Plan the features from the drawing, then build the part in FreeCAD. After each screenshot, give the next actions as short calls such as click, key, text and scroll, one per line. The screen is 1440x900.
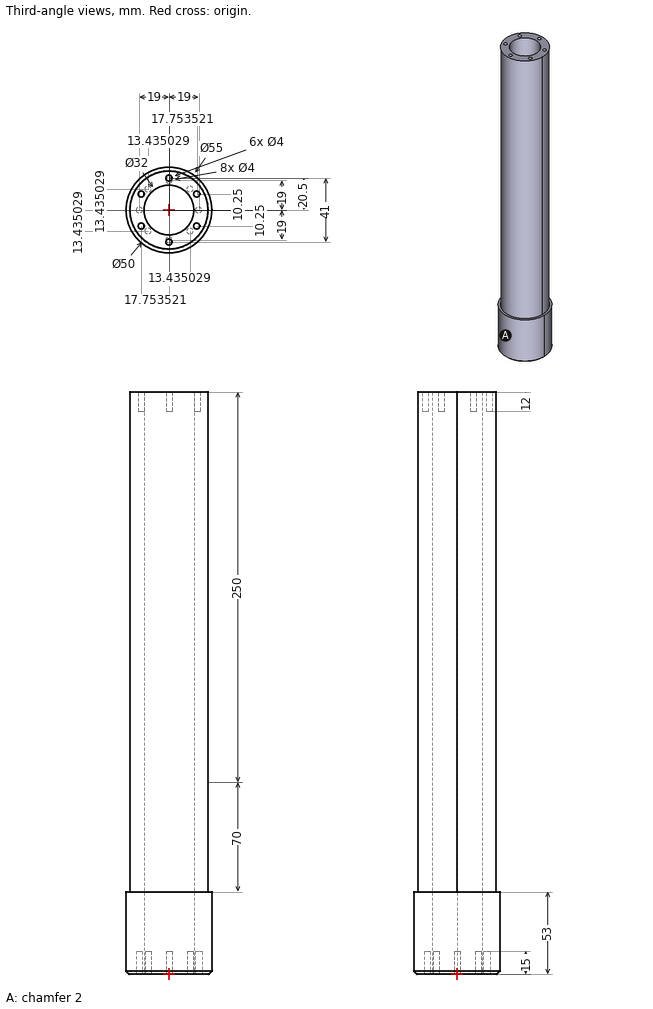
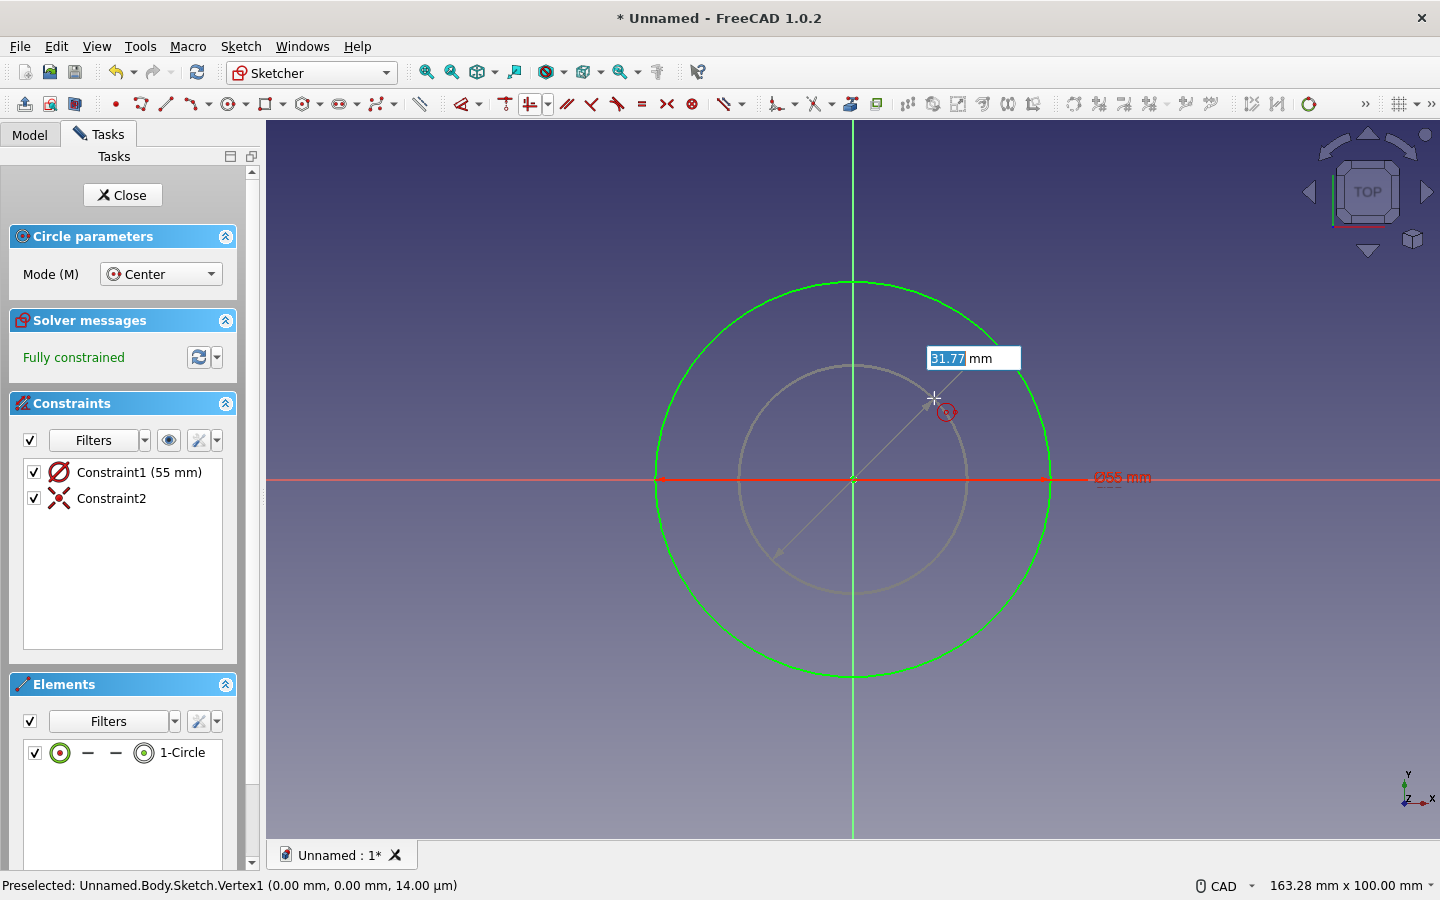
text(32)
key(Return)
key(Escape)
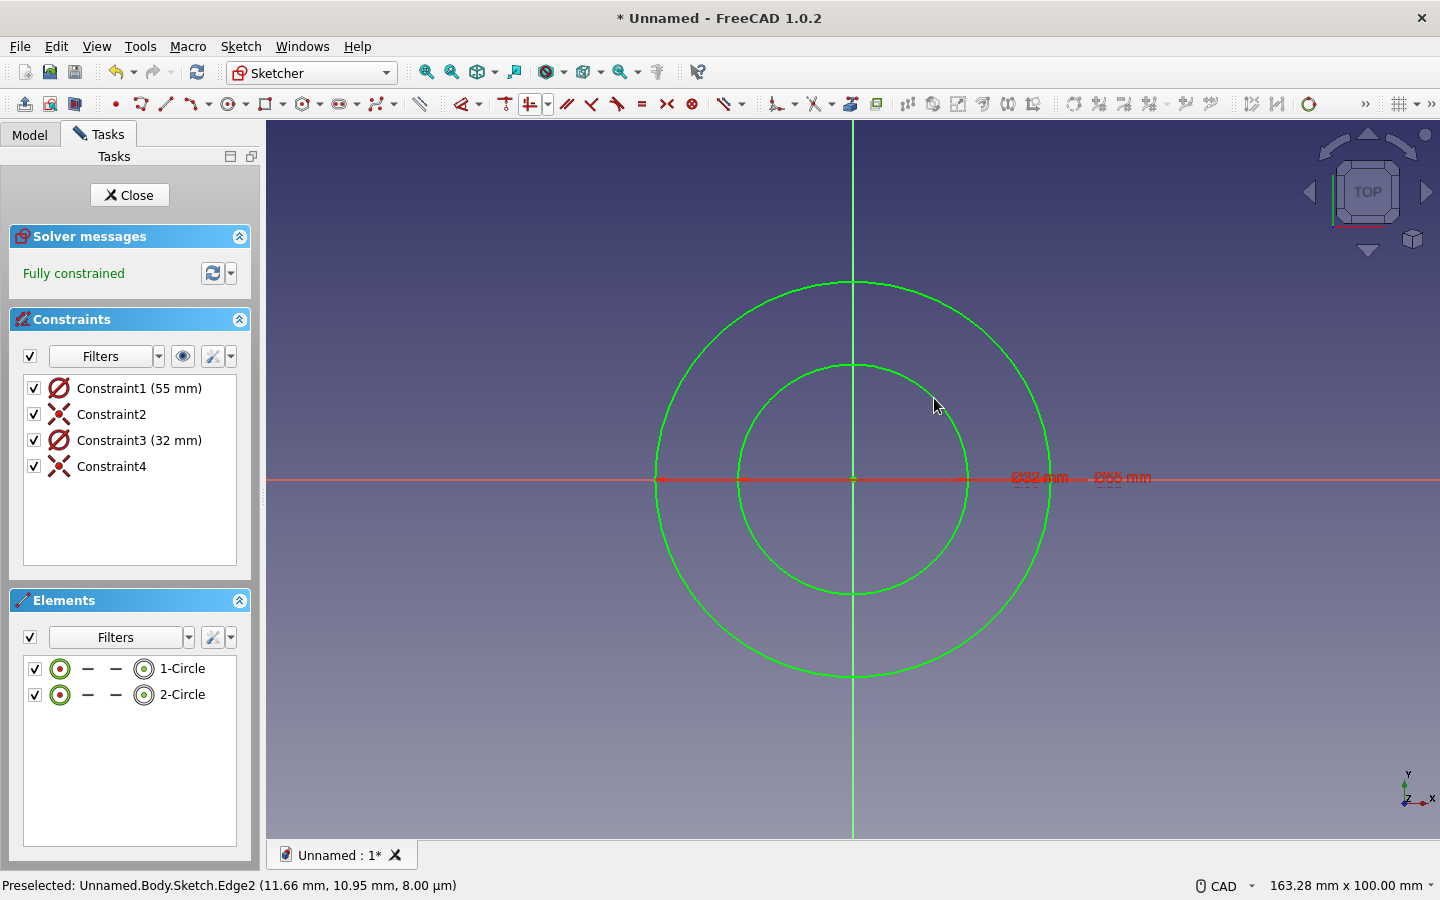
click(130, 195)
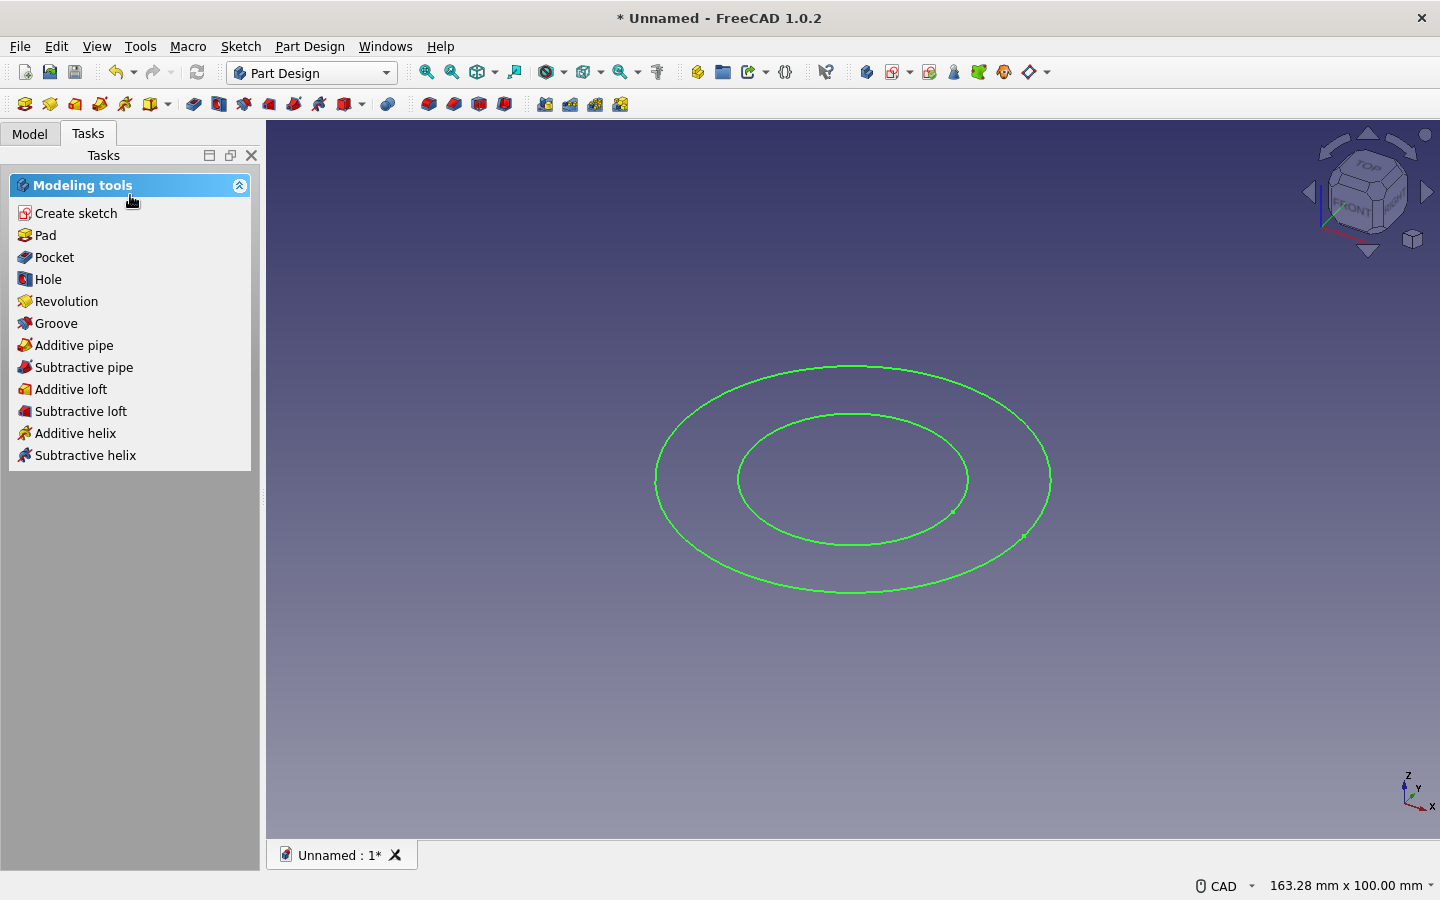
click(25, 104)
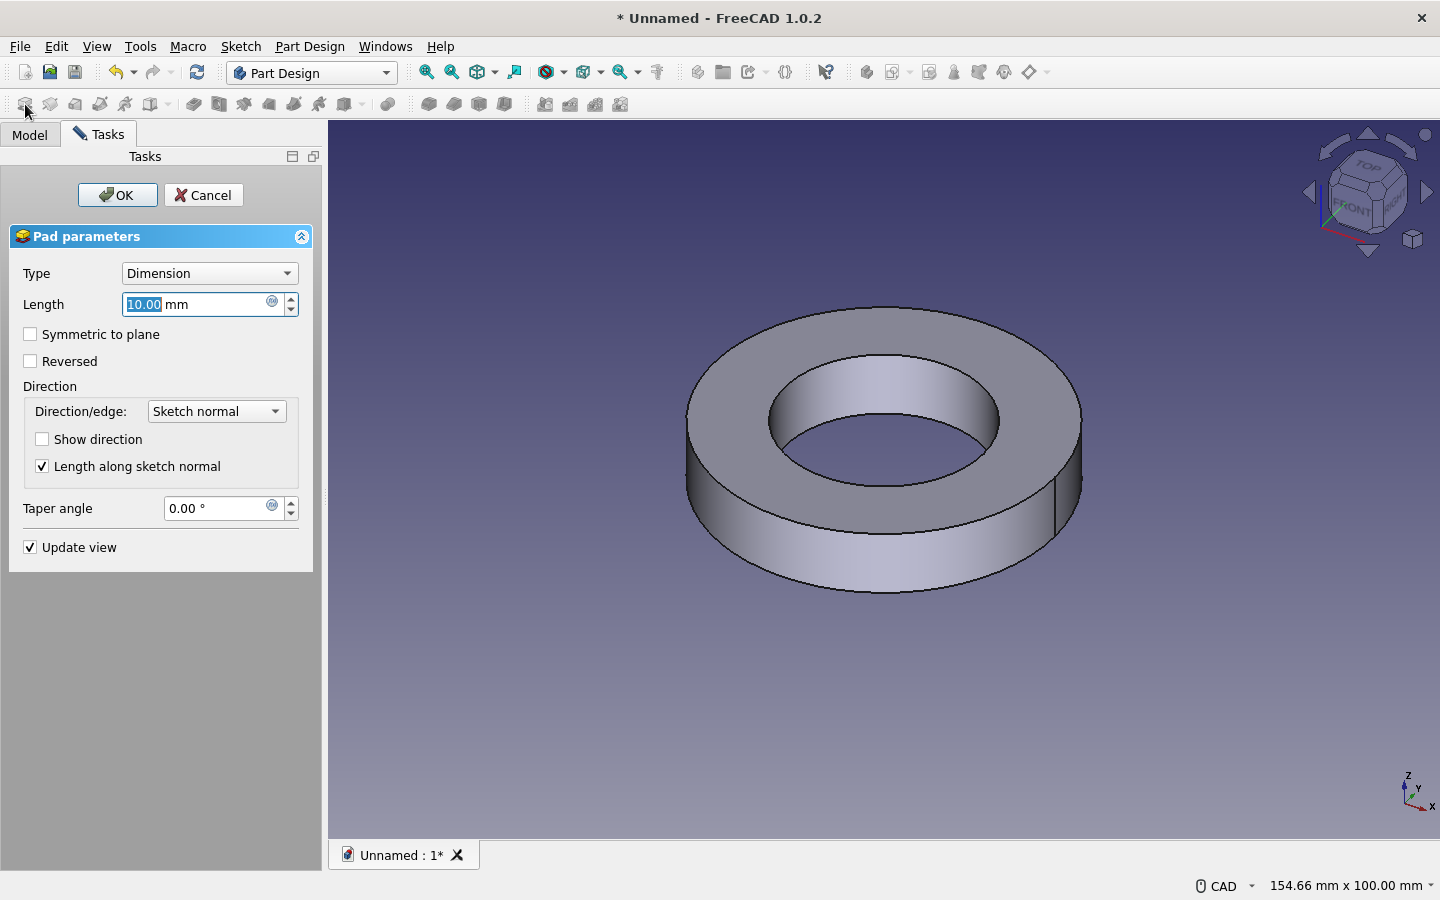
text(53)
key(Tab)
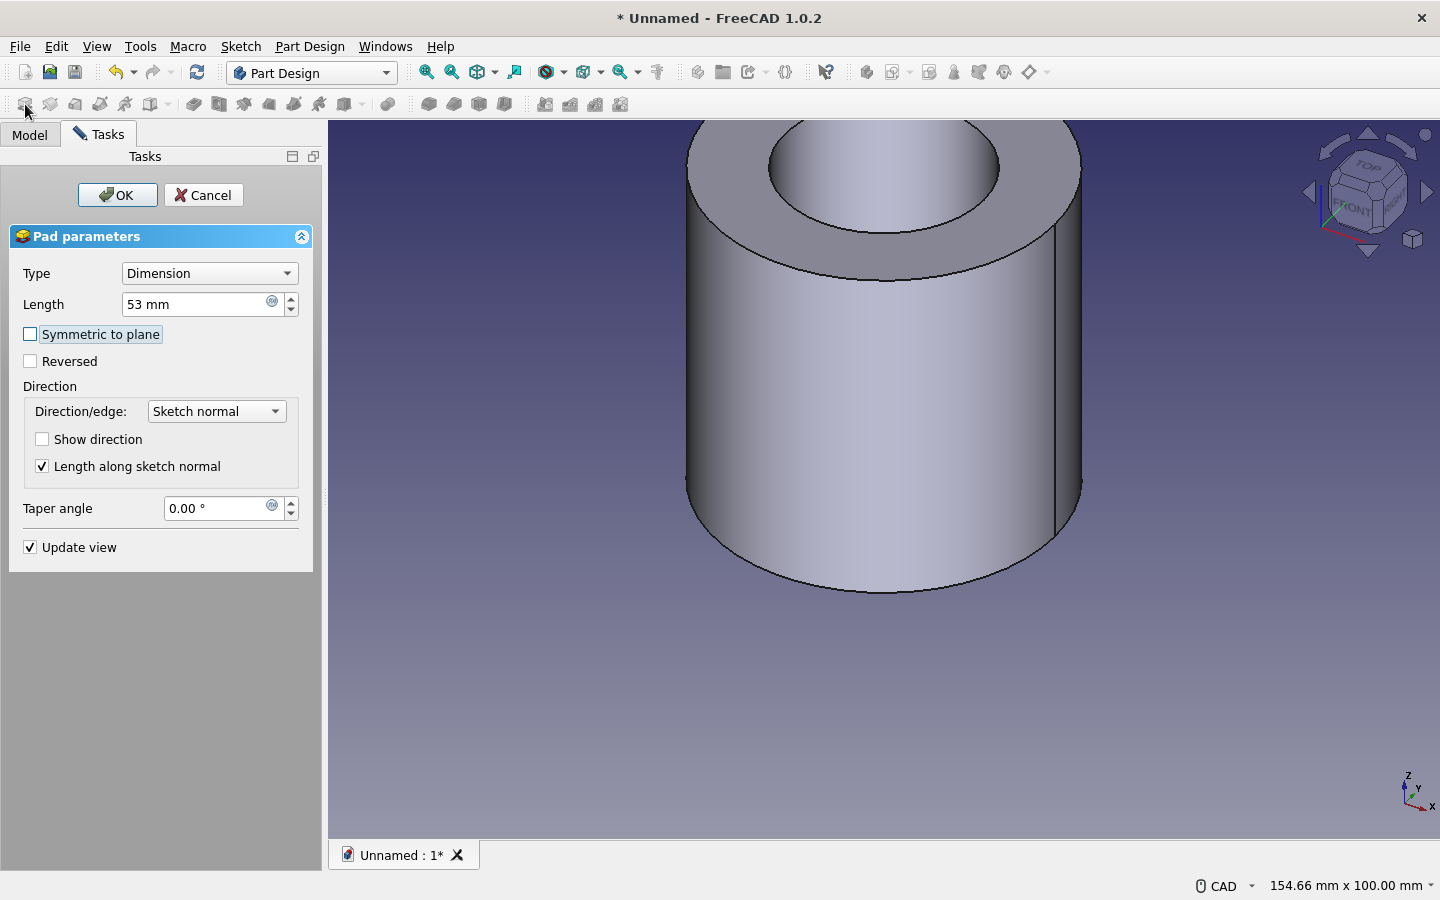
click(118, 195)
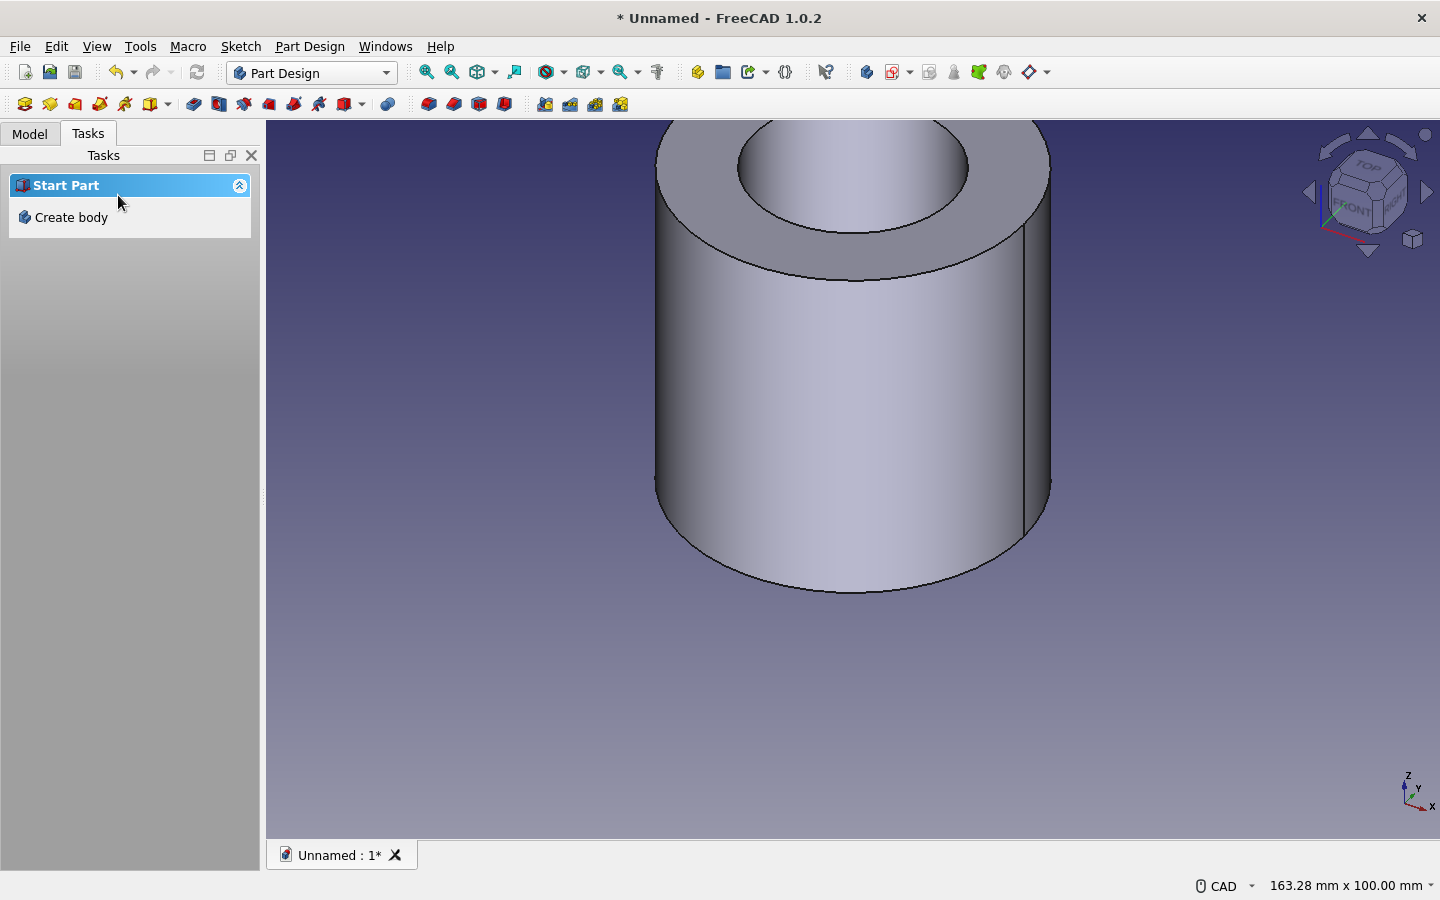
click(427, 72)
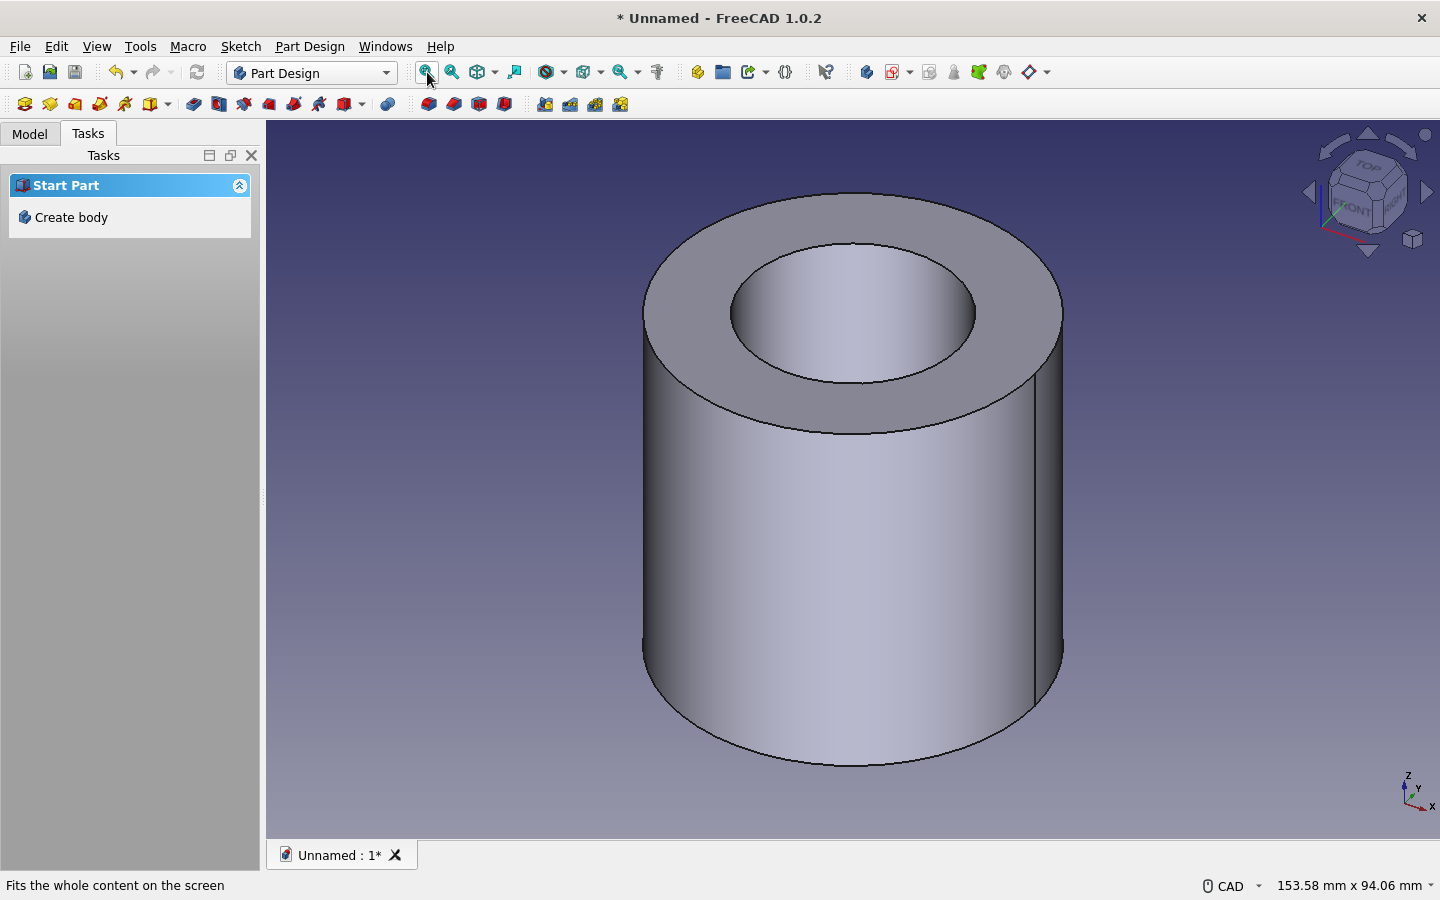
click(689, 338)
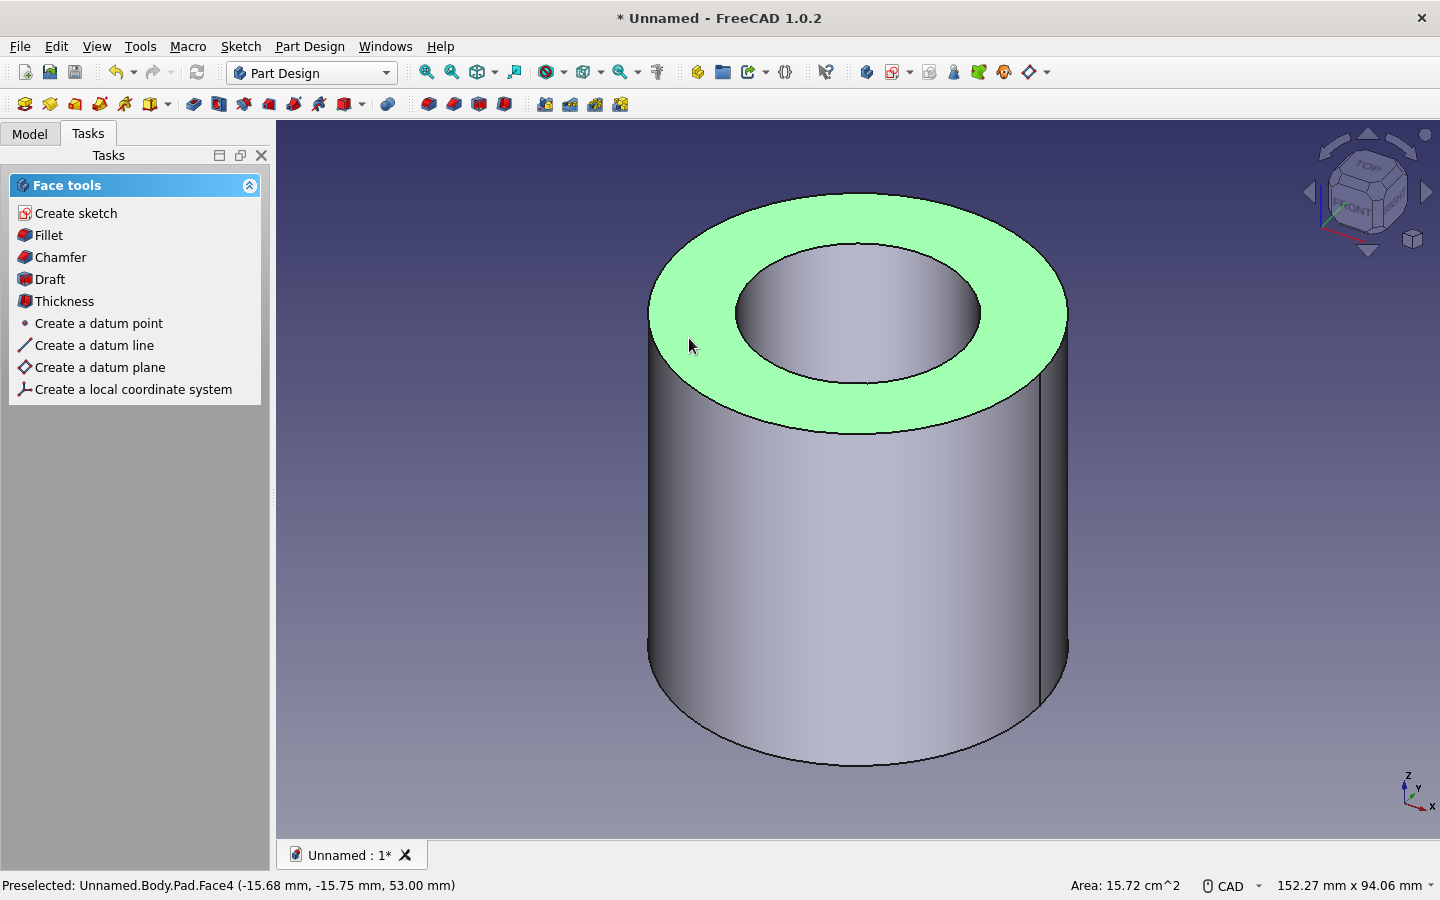
click(892, 72)